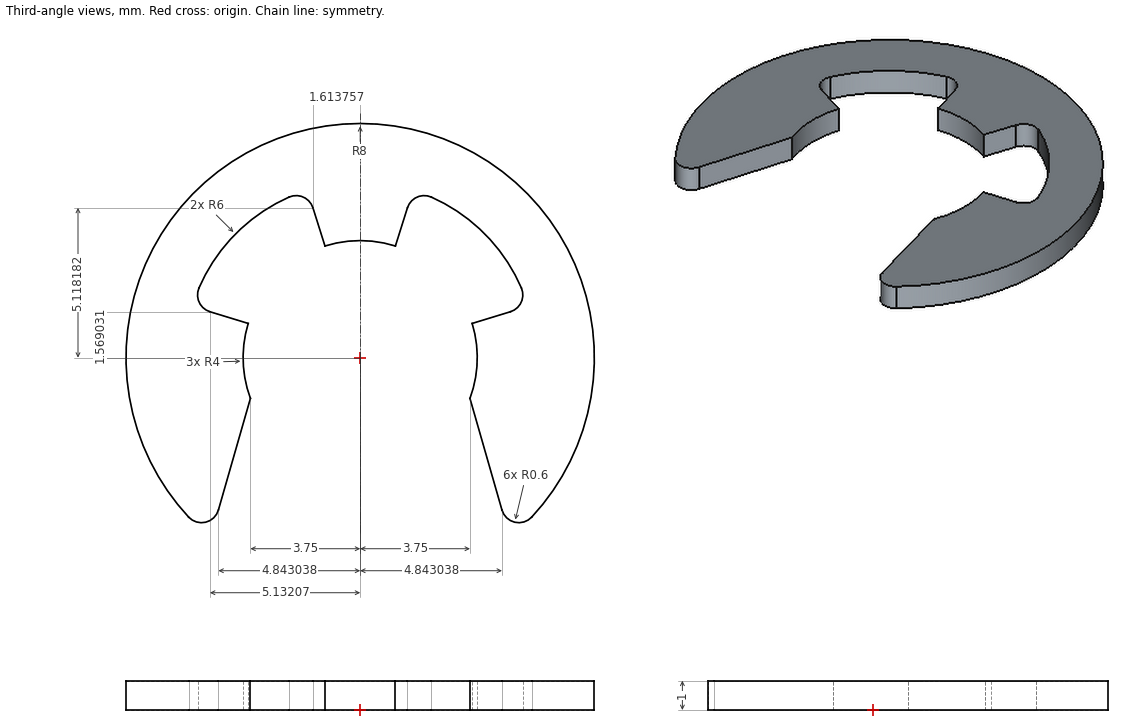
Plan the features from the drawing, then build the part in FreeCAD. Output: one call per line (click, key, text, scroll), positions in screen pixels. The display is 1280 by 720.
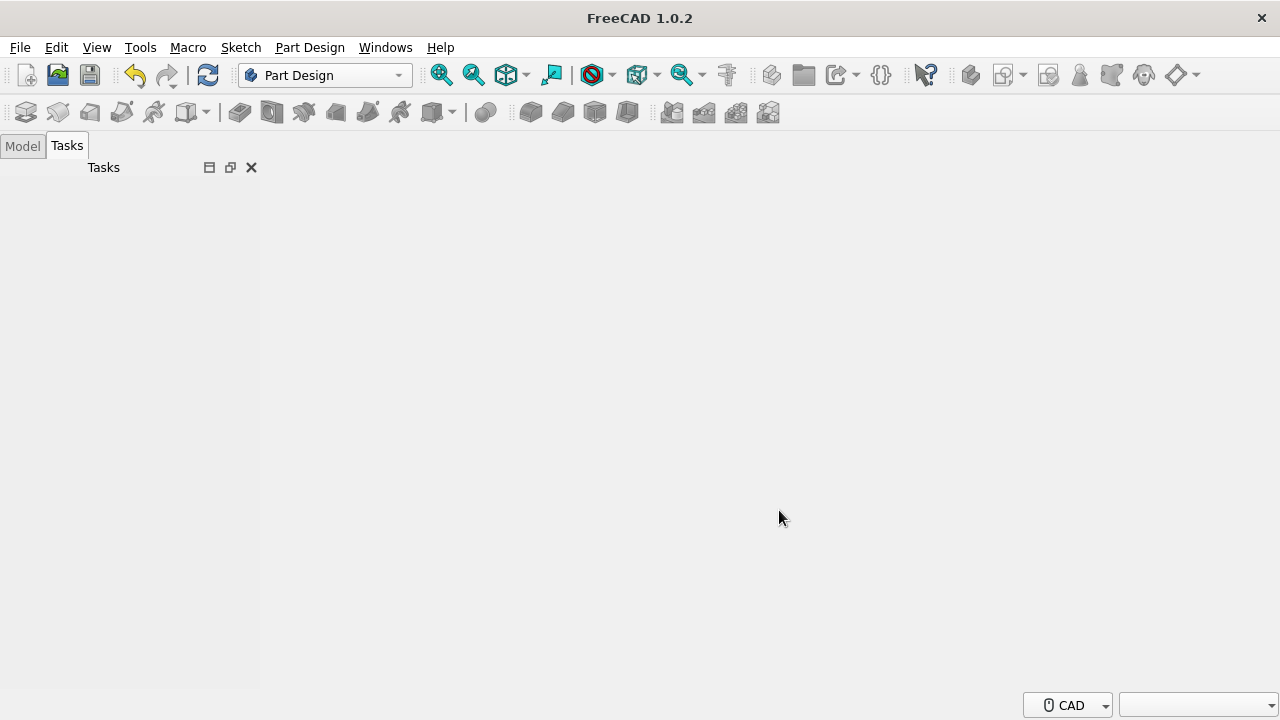
key(ctrl+n)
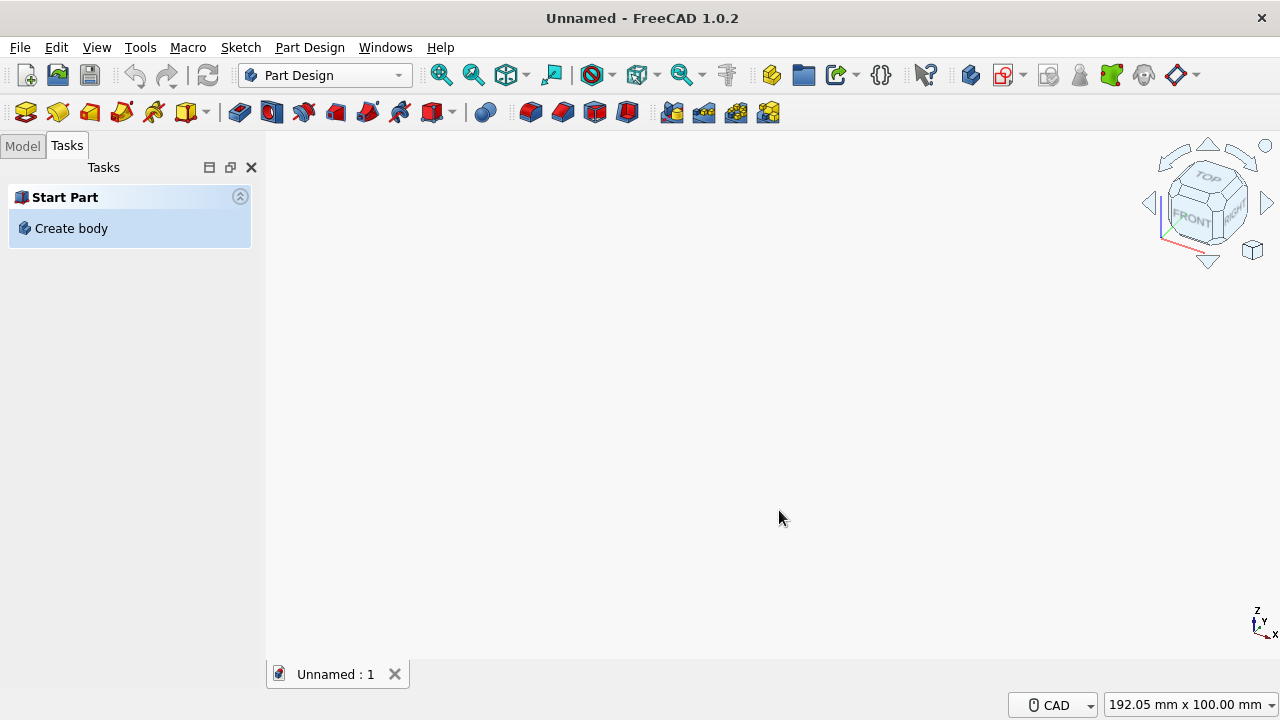
click(1004, 76)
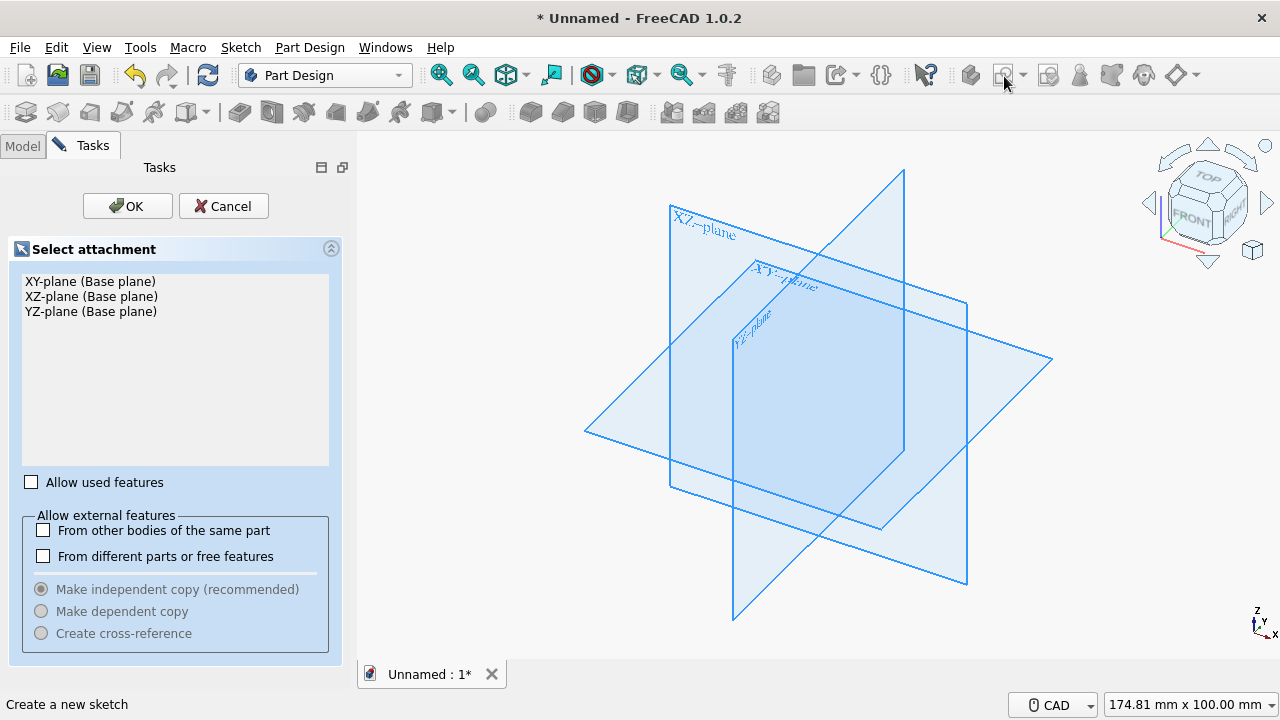
click(82, 282)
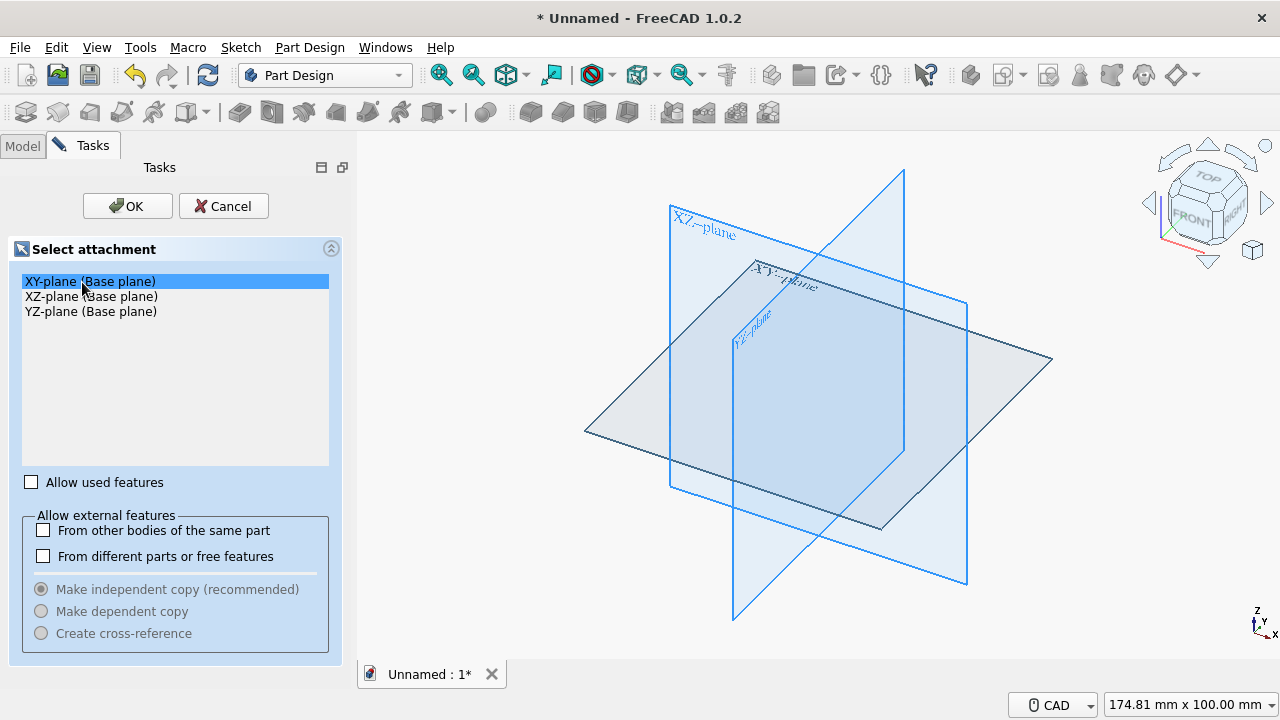
click(128, 206)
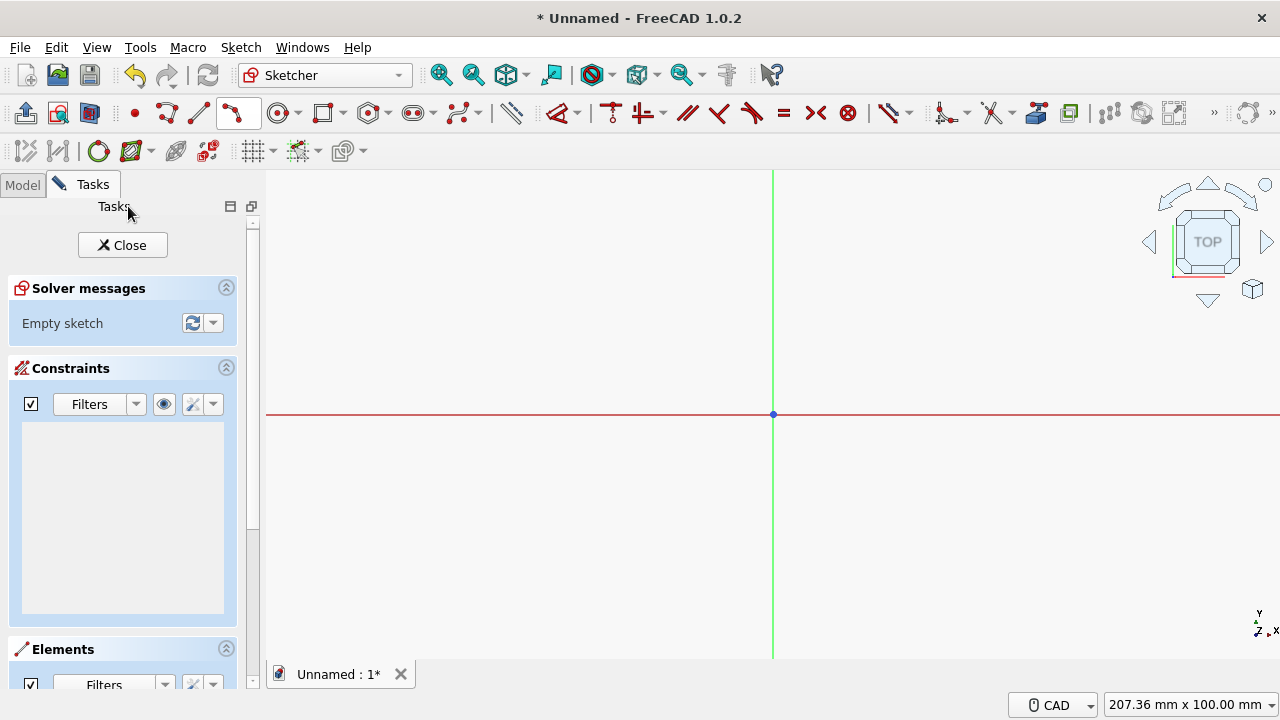
scroll(790, 407, up, 8)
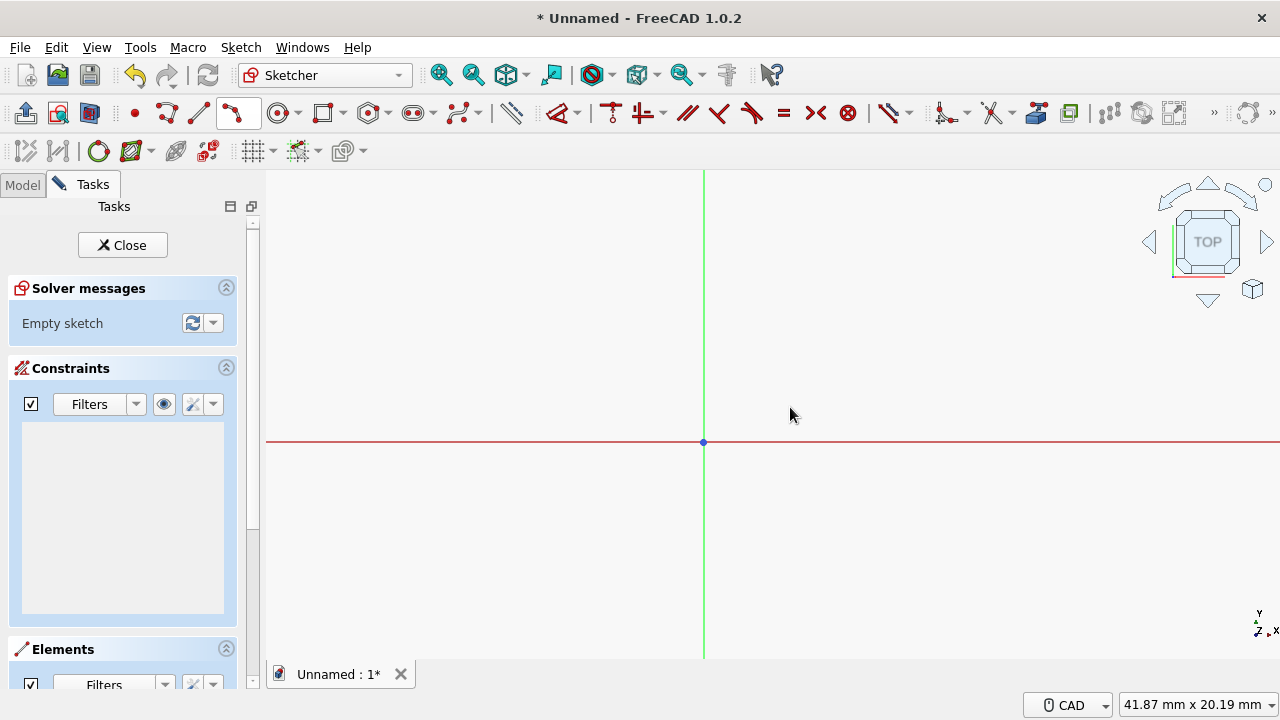
click(200, 114)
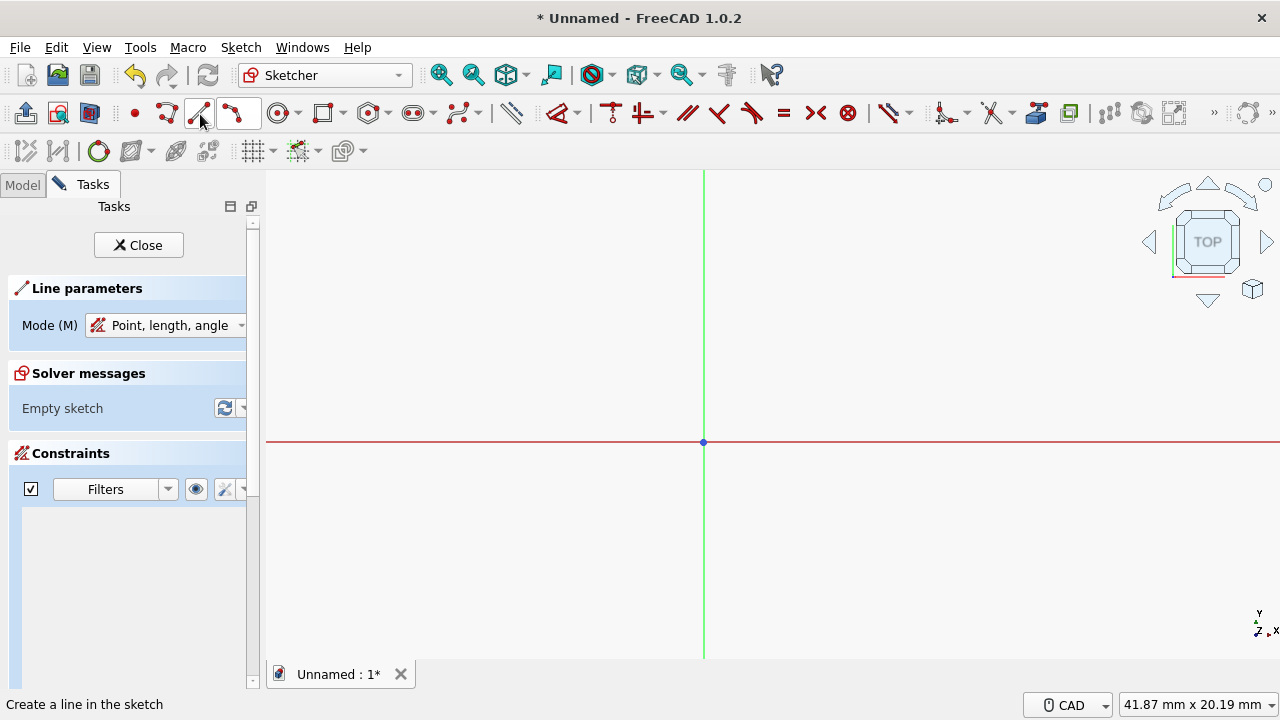
click(795, 476)
click(821, 568)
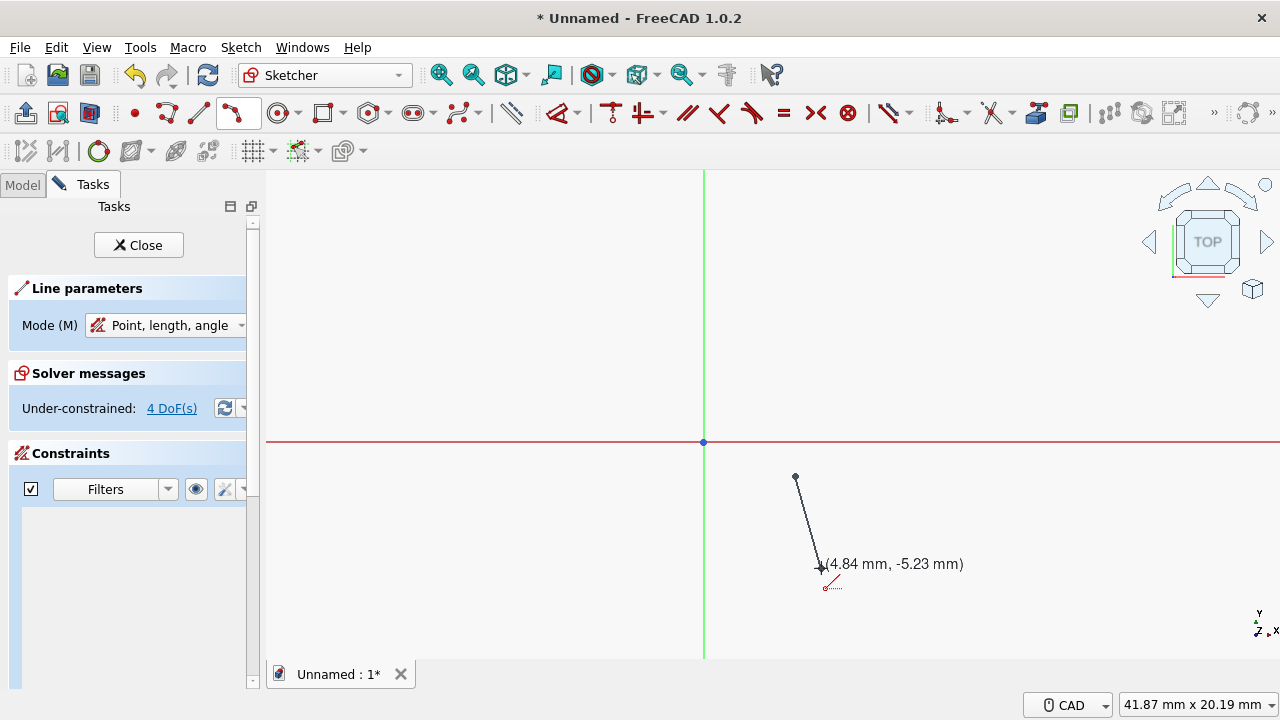
click(586, 568)
click(613, 476)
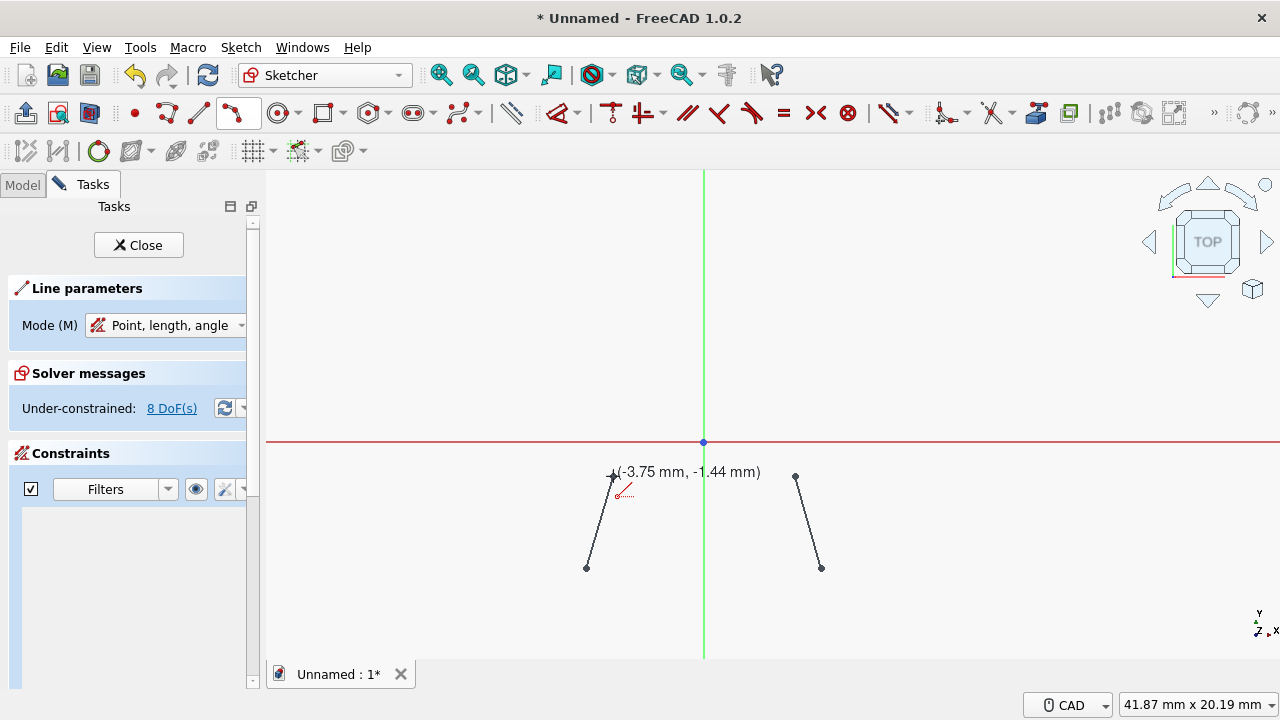
click(611, 414)
click(579, 404)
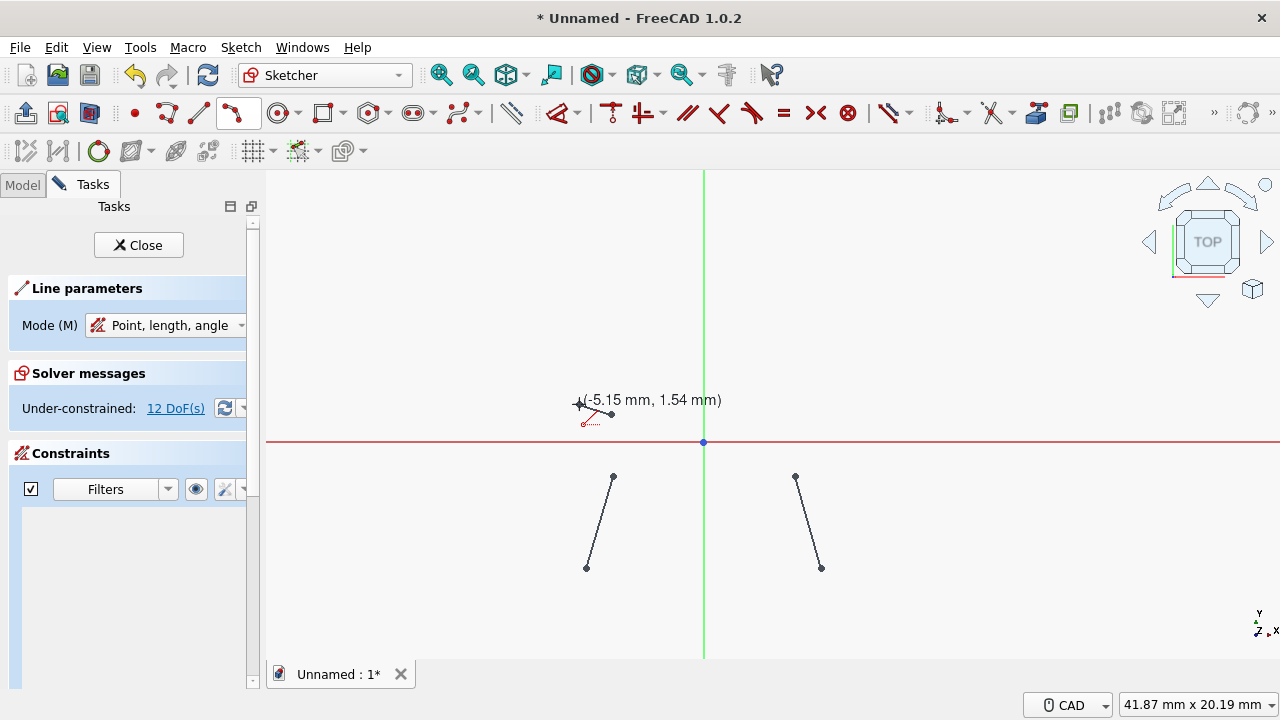
click(665, 318)
click(675, 350)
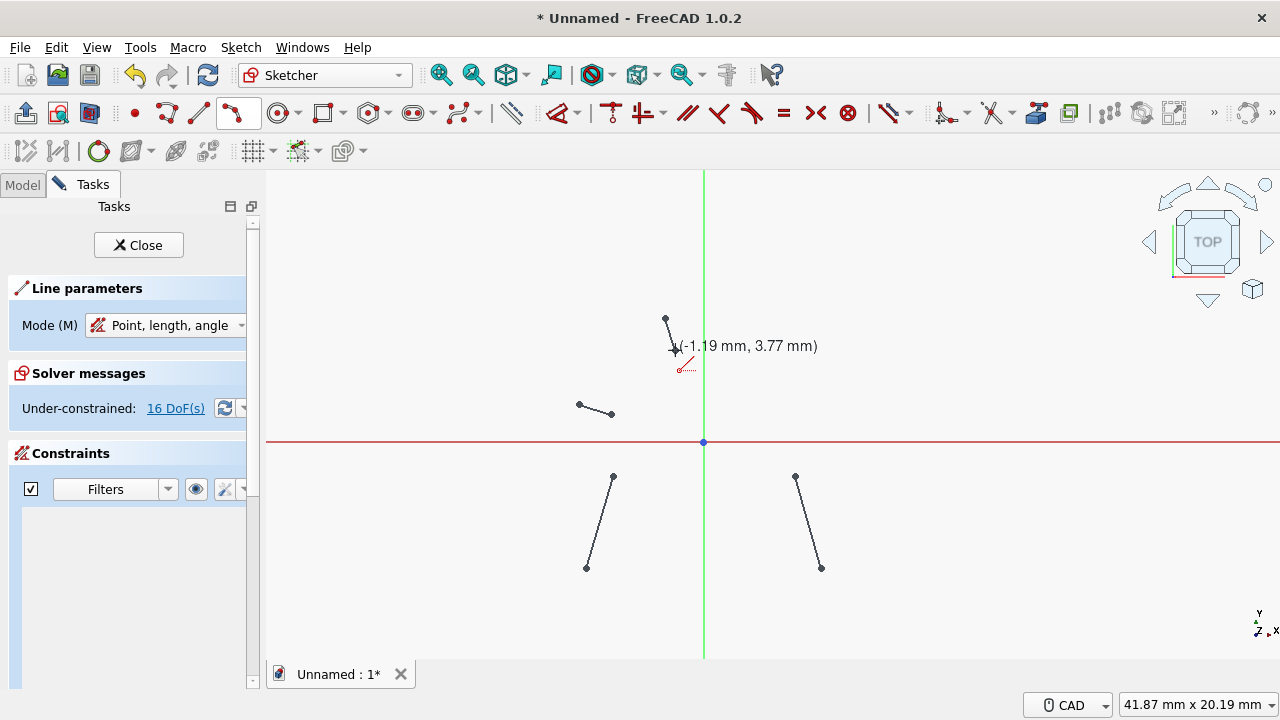
click(733, 350)
click(743, 318)